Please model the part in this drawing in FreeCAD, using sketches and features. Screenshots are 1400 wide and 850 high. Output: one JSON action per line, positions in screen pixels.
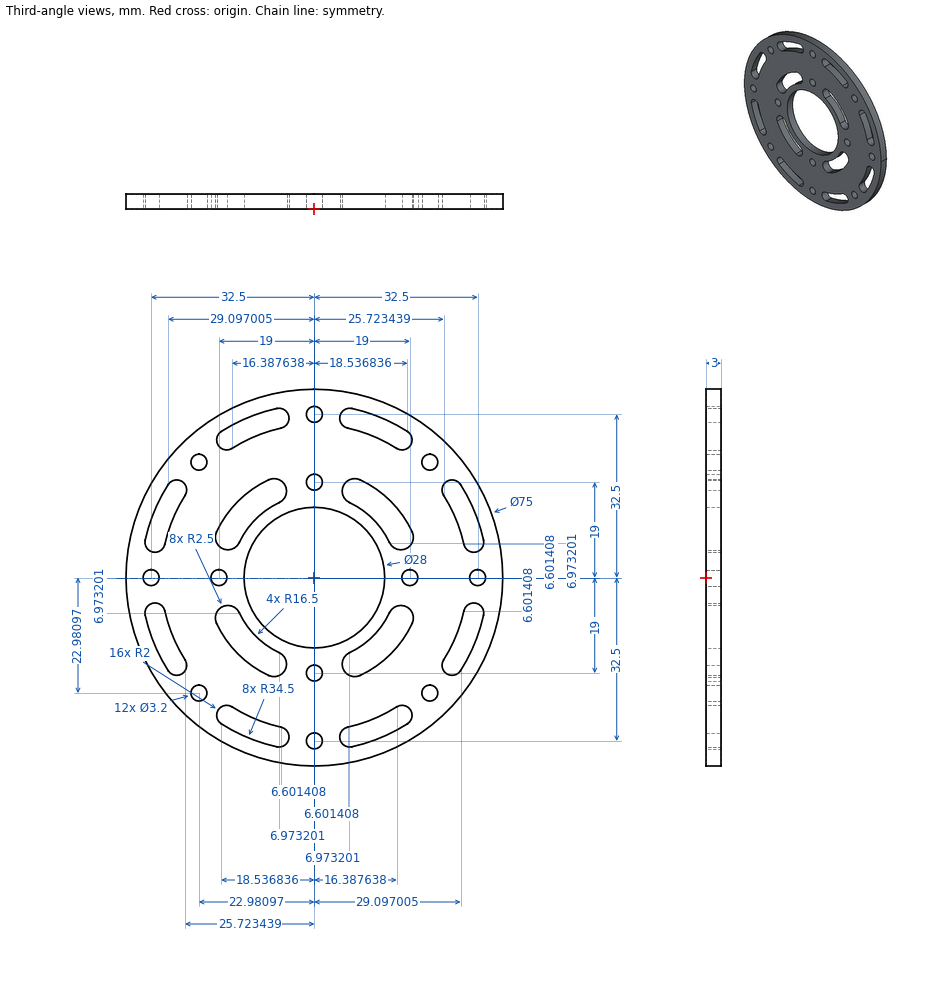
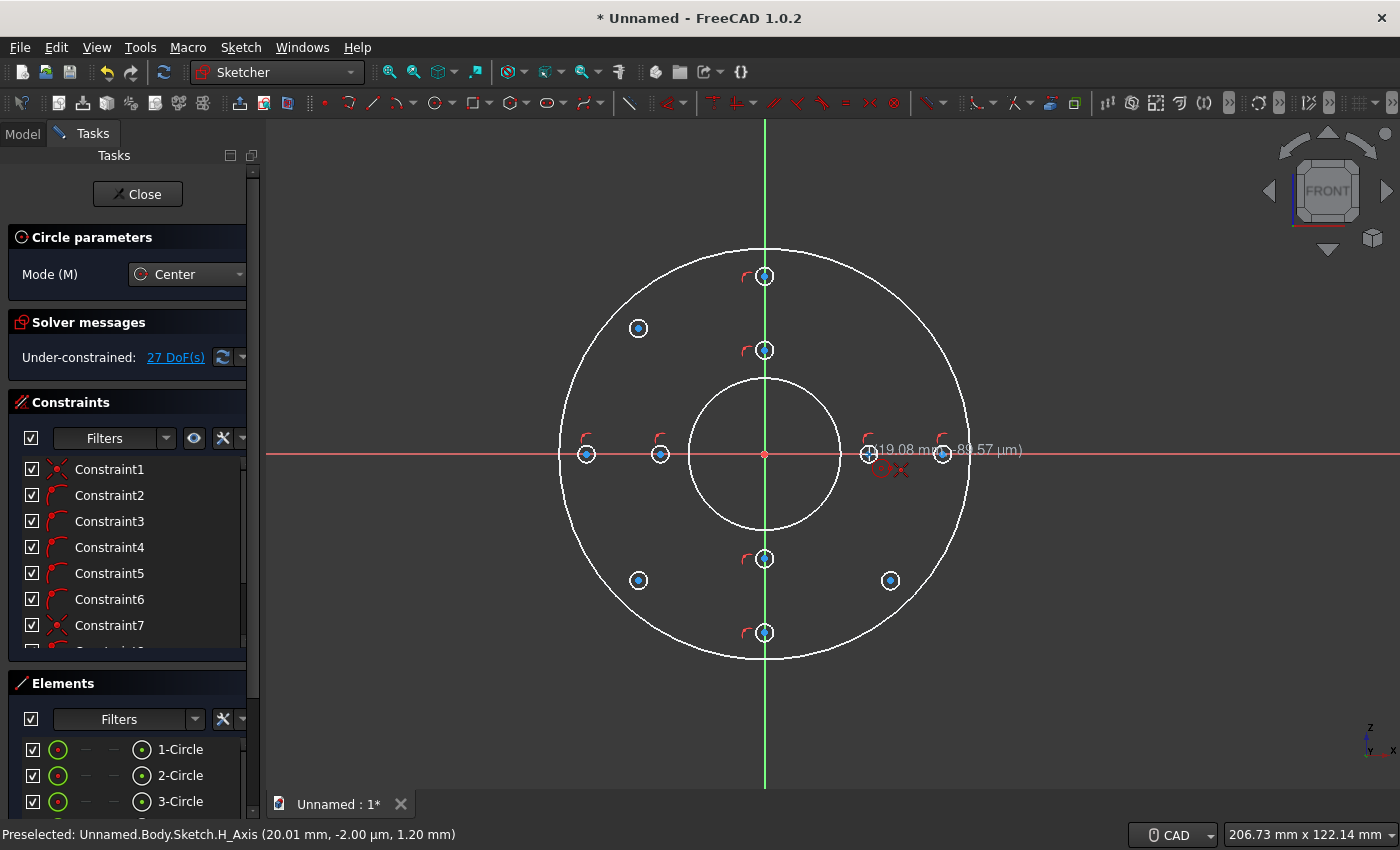
{"action": "scroll", "coordinate": [891, 328], "scroll_direction": "up", "scroll_amount": 5}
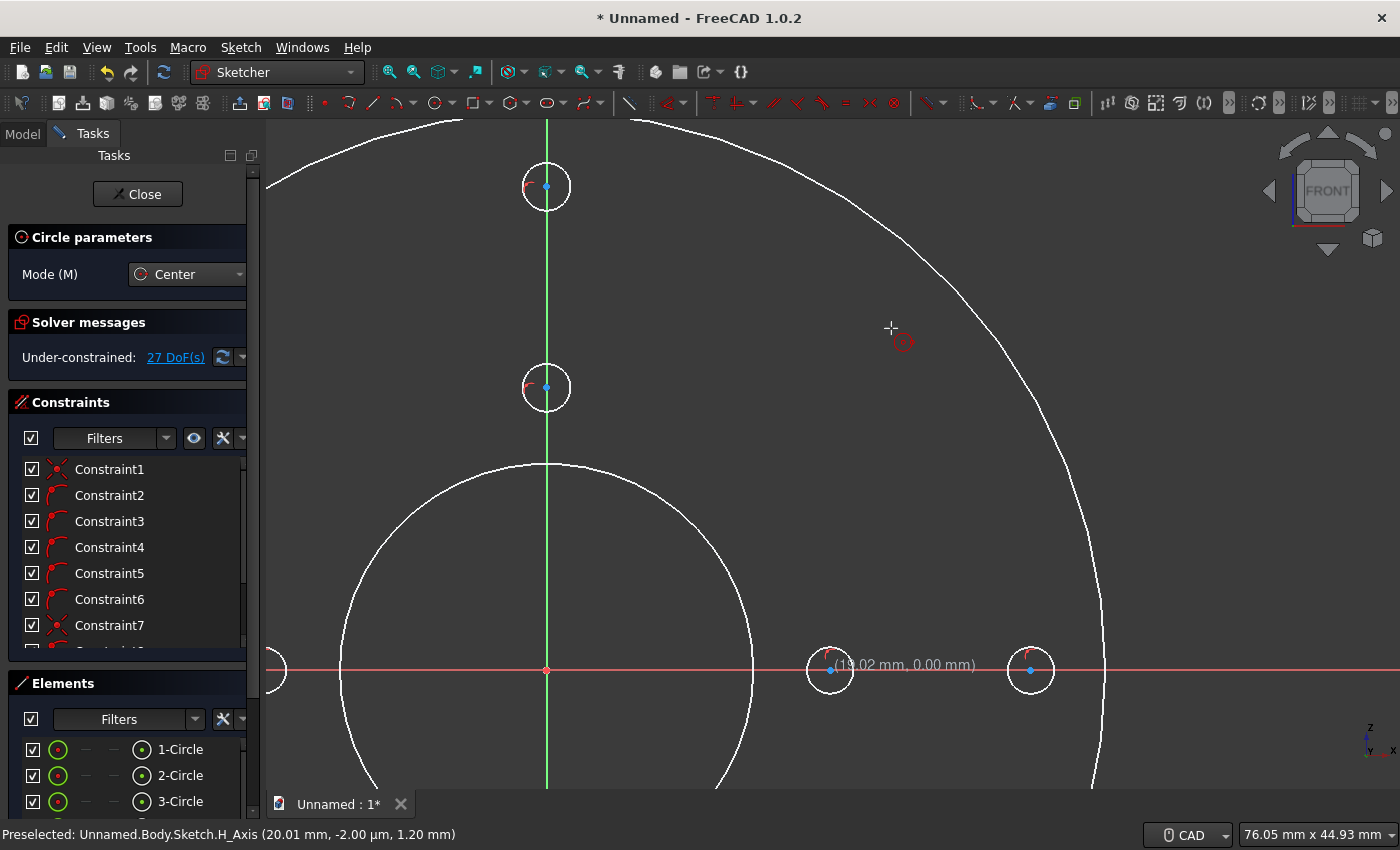
{"action": "left_click", "coordinate": [889, 328]}
{"action": "left_click", "coordinate": [906, 311]}
{"action": "key", "text": "Escape"}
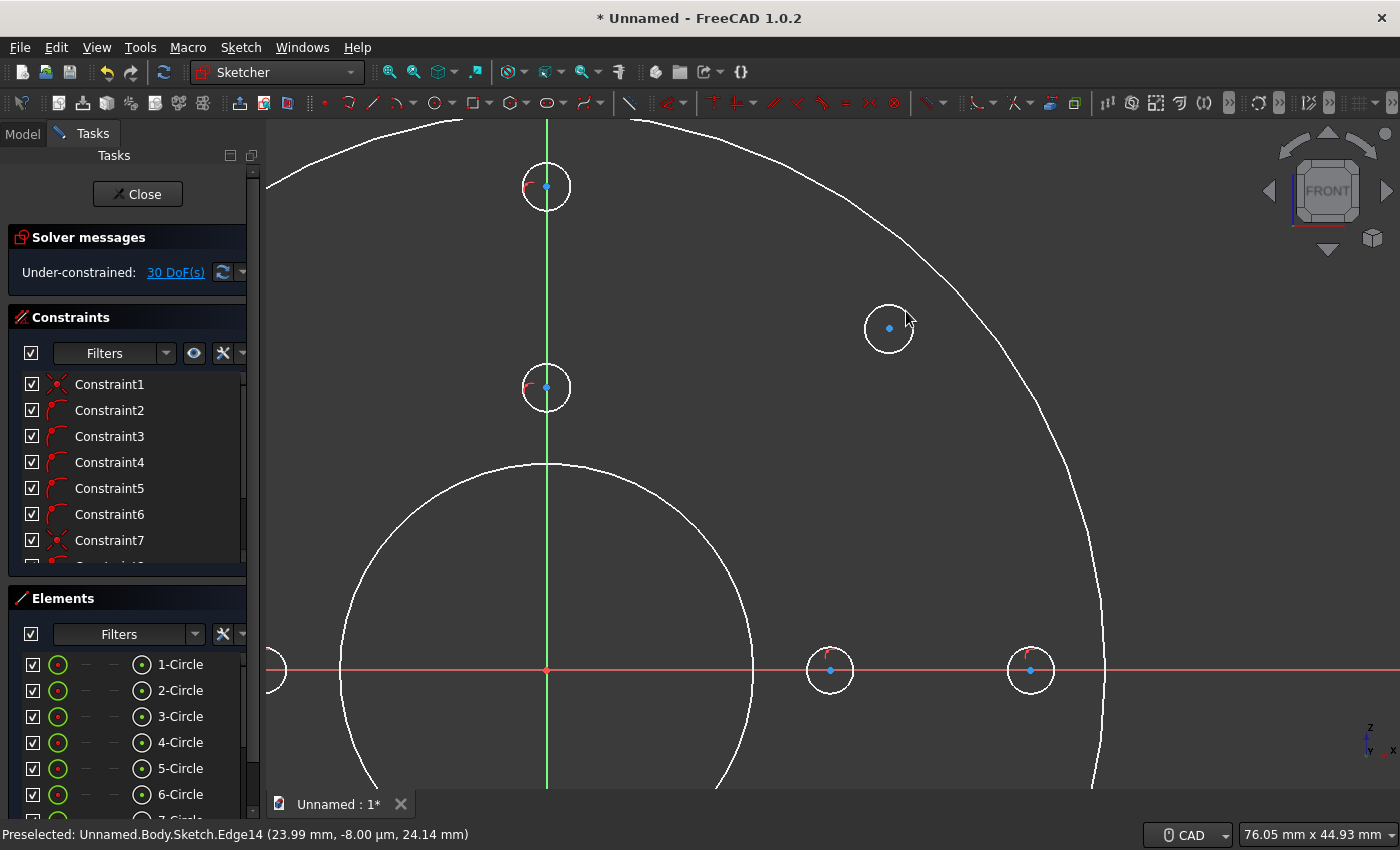
{"action": "scroll", "coordinate": [891, 328], "scroll_direction": "down", "scroll_amount": 5}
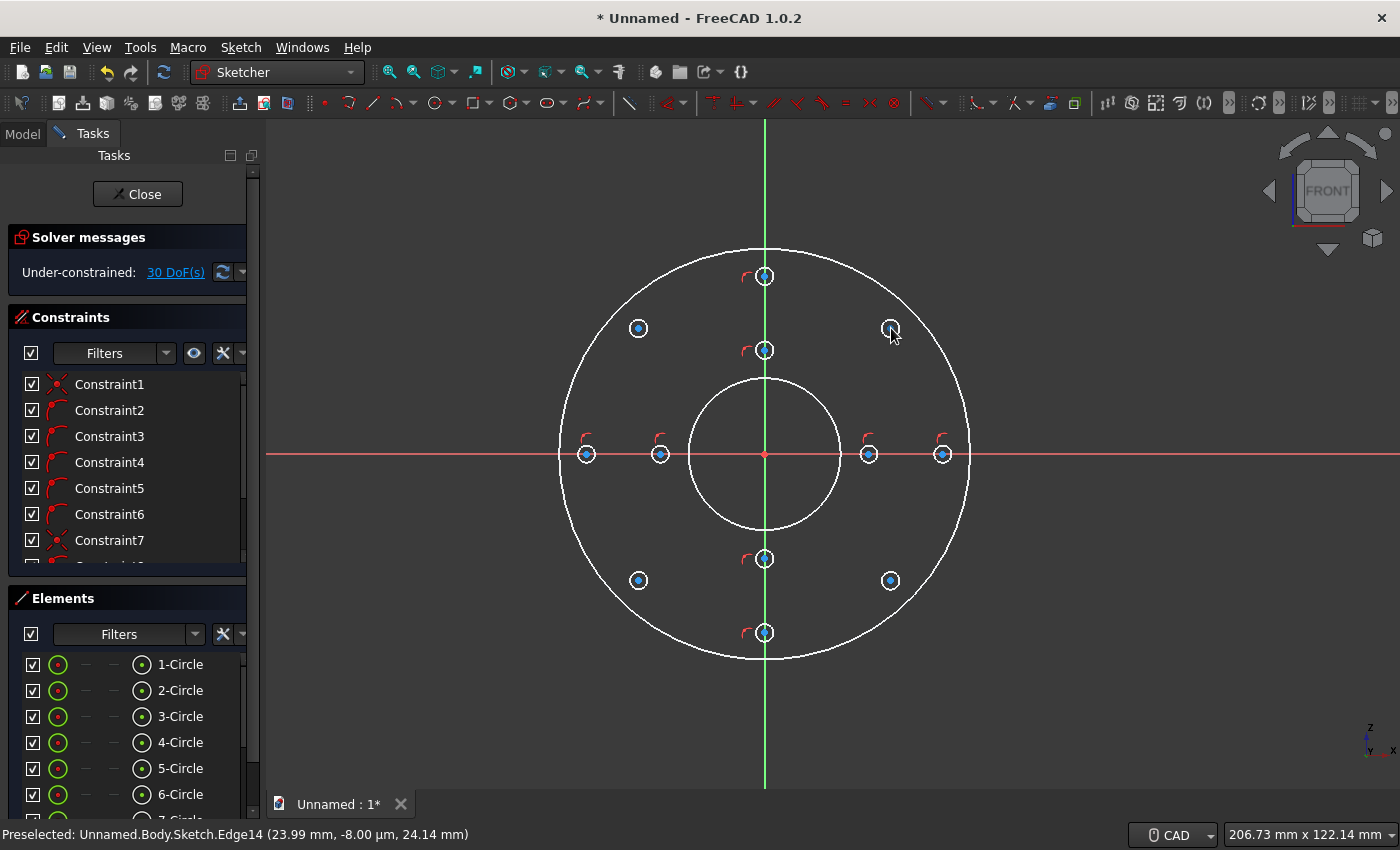
{"action": "scroll", "coordinate": [645, 575], "scroll_direction": "up", "scroll_amount": 3}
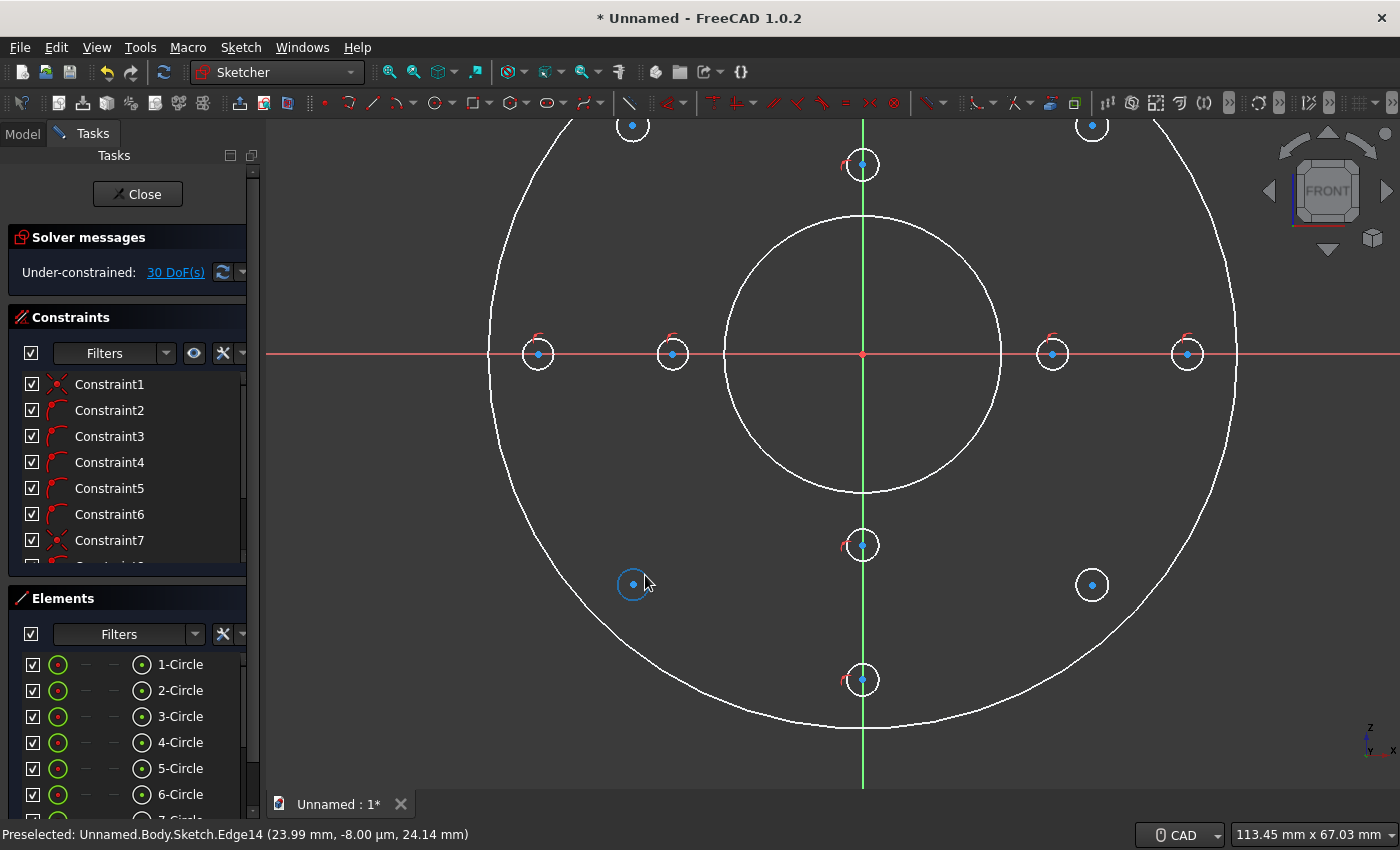
{"action": "left_click", "coordinate": [644, 574]}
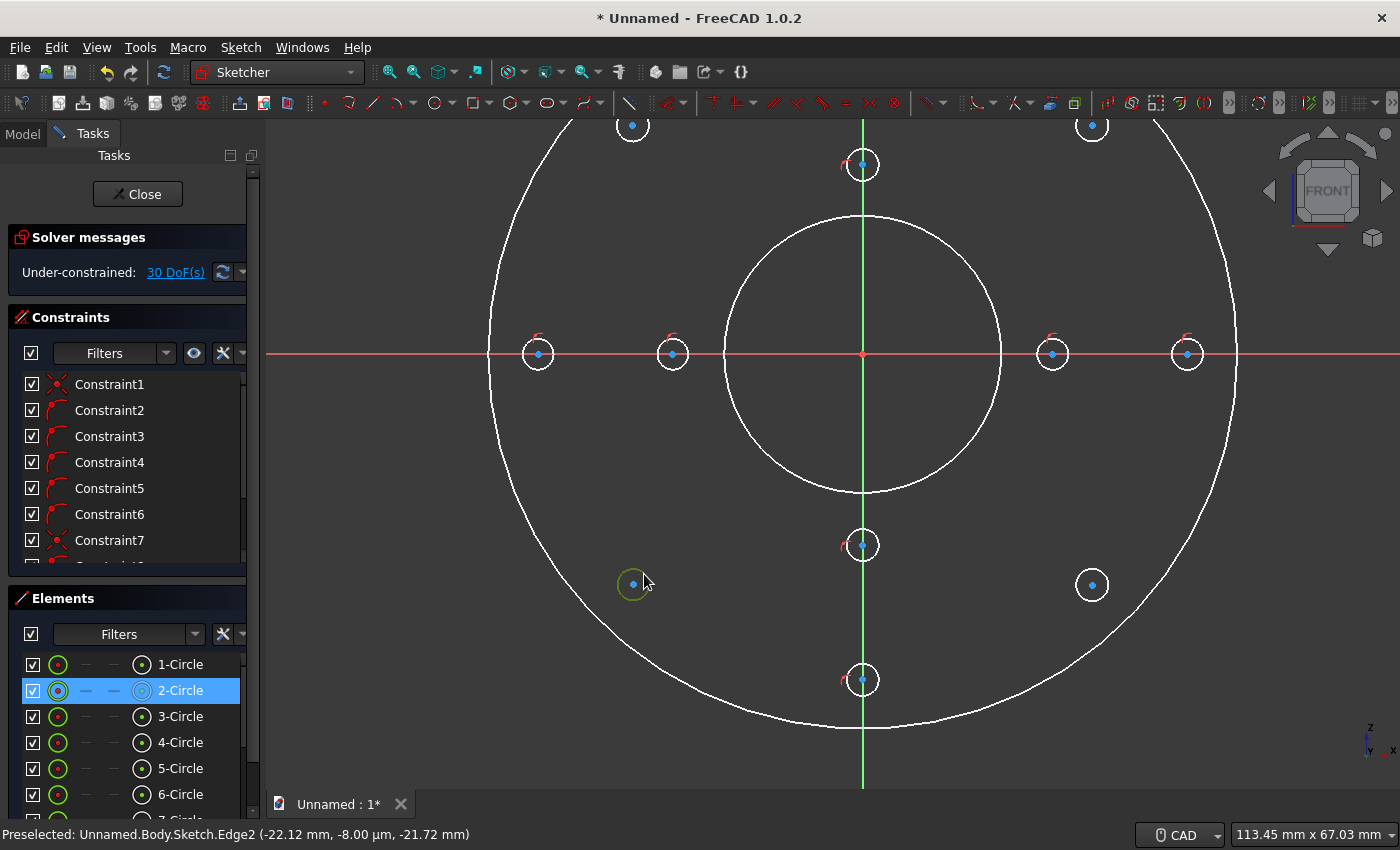
{"action": "scroll", "coordinate": [874, 669], "scroll_direction": "up", "scroll_amount": 2}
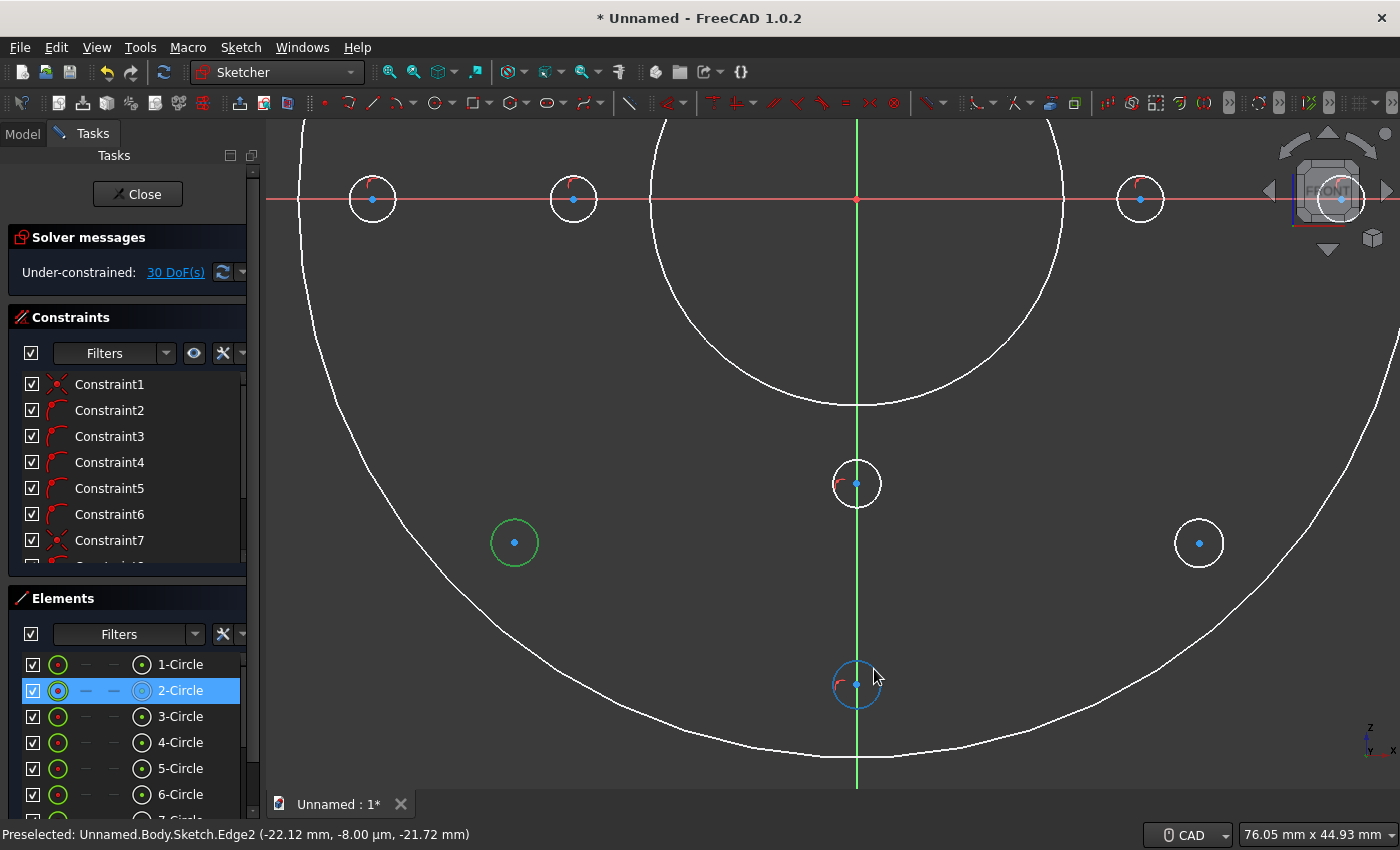
{"action": "left_click", "coordinate": [874, 668]}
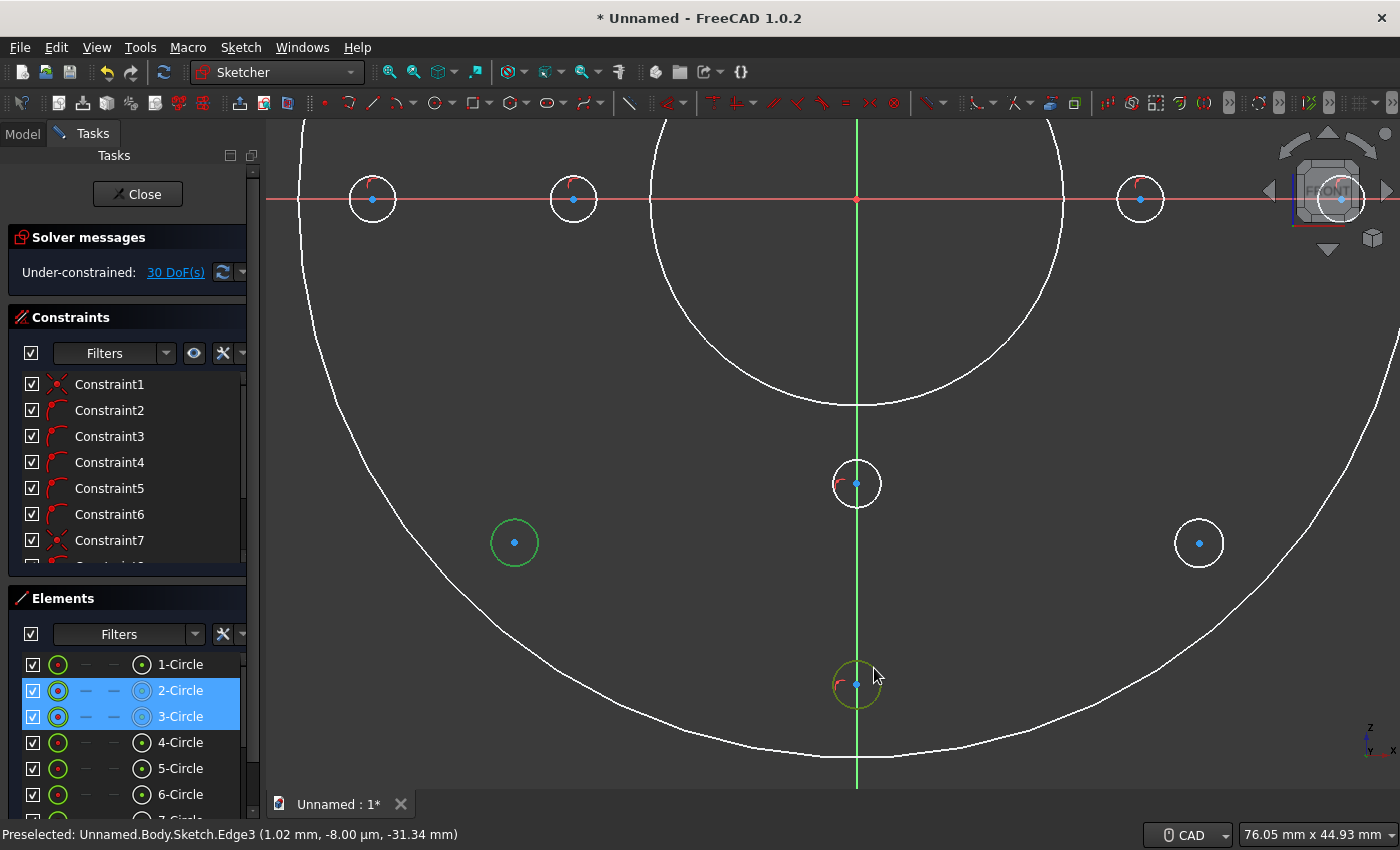
{"action": "left_click", "coordinate": [874, 467]}